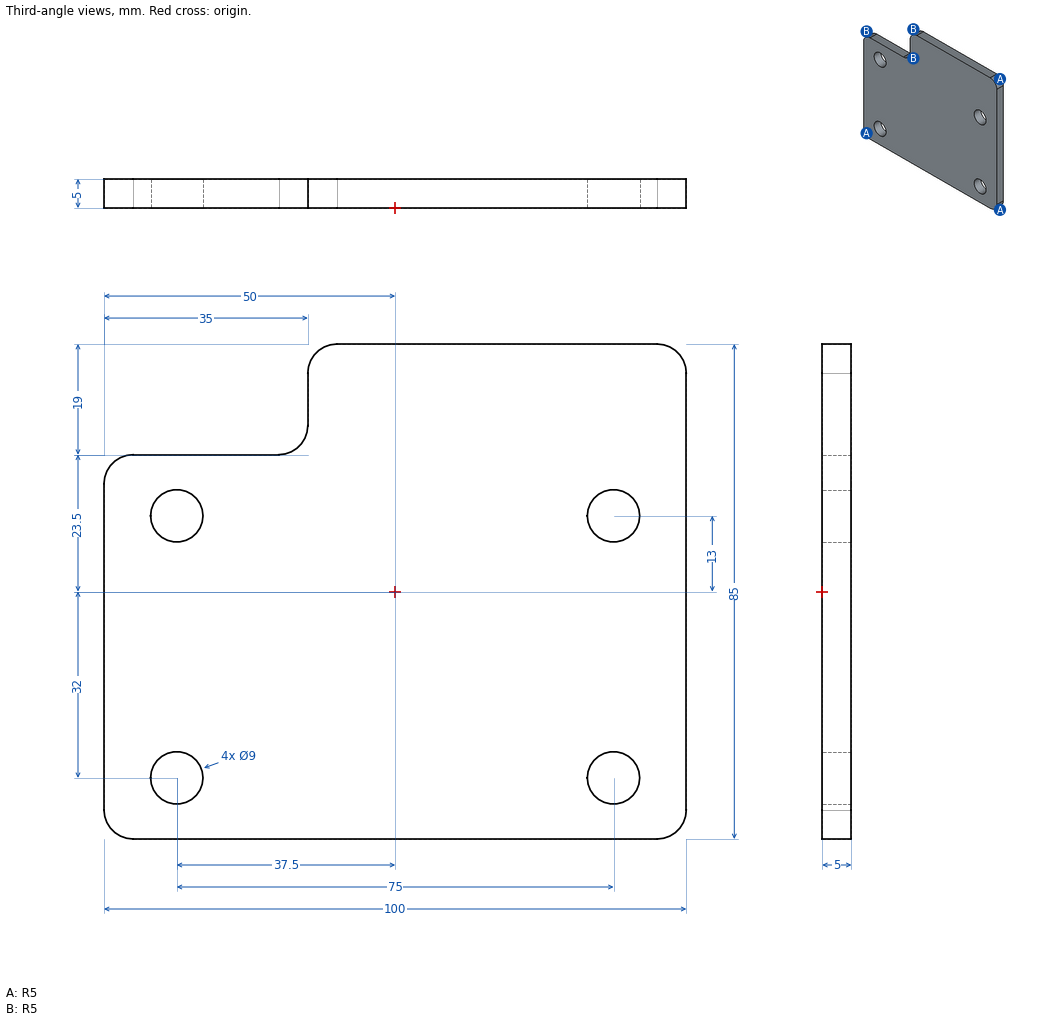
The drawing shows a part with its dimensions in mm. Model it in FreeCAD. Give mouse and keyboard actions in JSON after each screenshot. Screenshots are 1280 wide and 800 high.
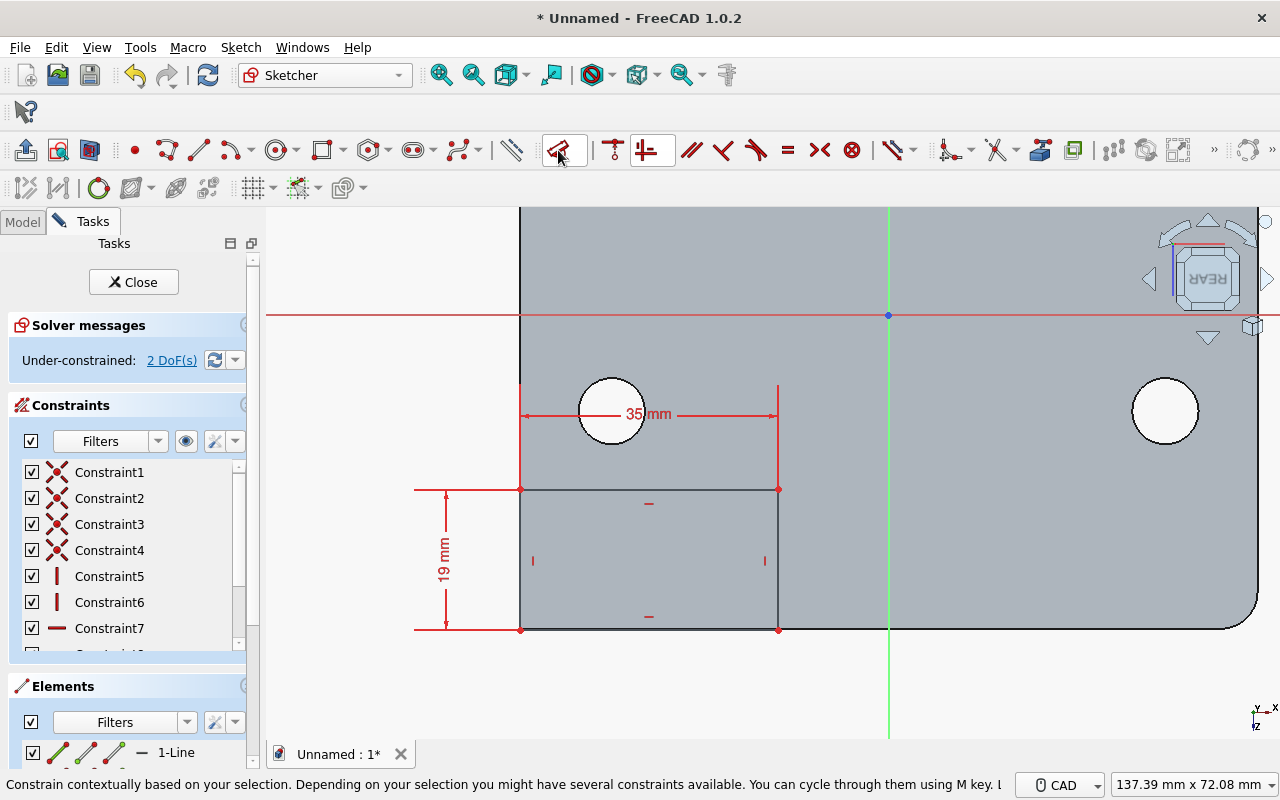
{"action": "left_click", "coordinate": [520, 490]}
{"action": "left_click", "coordinate": [704, 281]}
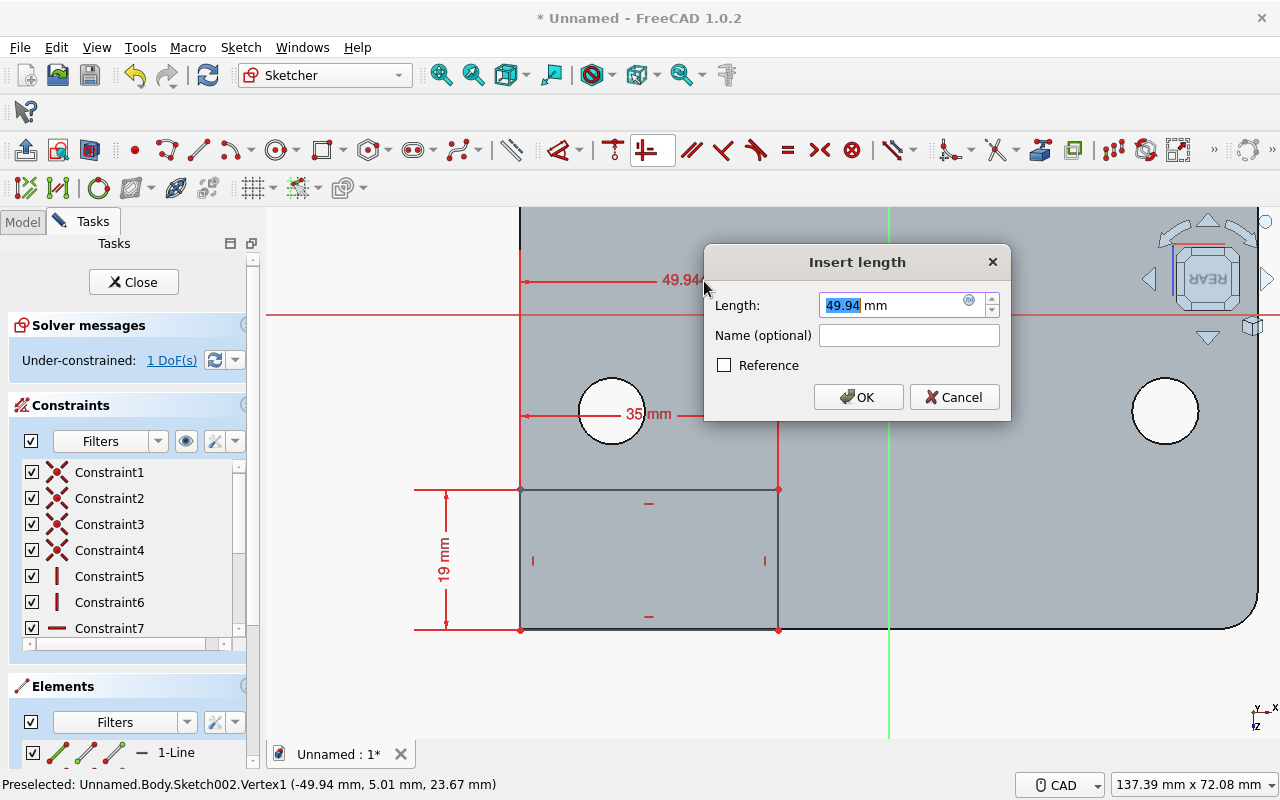
{"action": "type", "text": "50"}
{"action": "key", "text": "Return"}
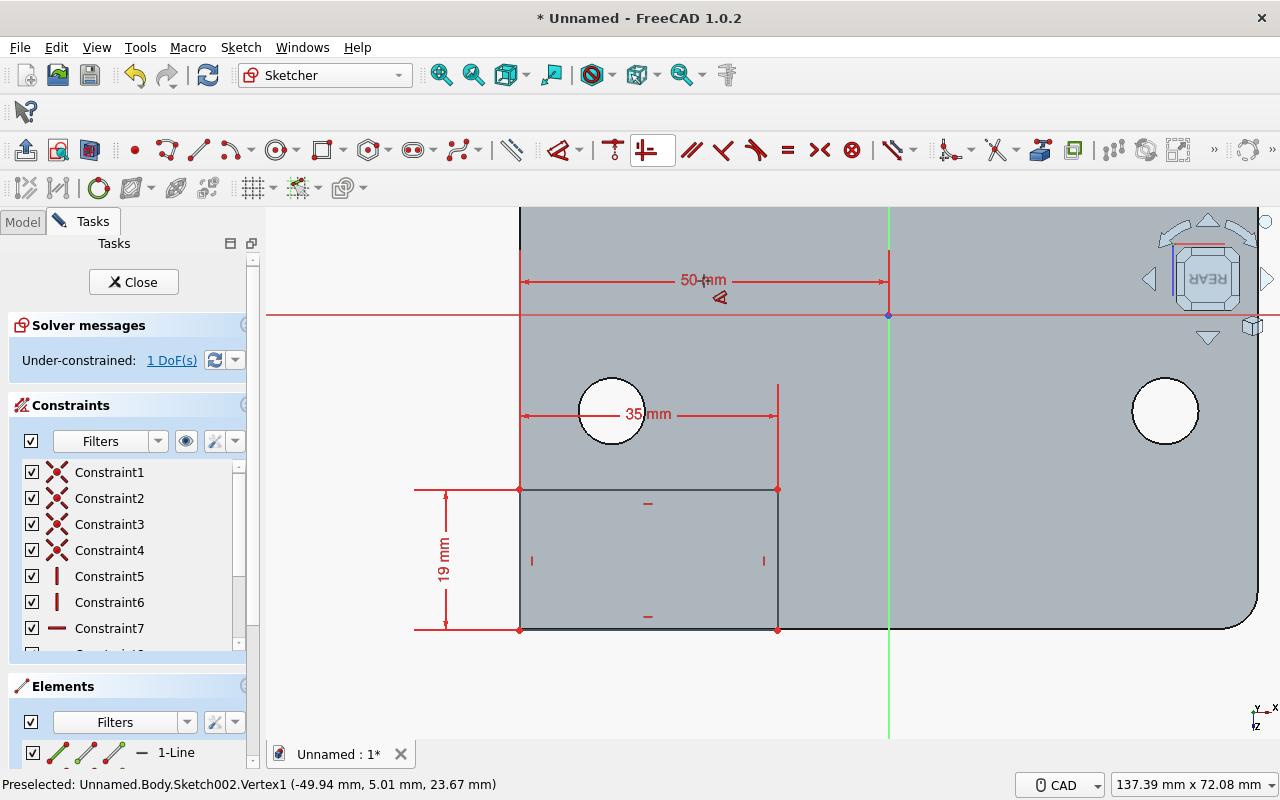
{"action": "left_click", "coordinate": [520, 490]}
{"action": "left_click", "coordinate": [923, 403]}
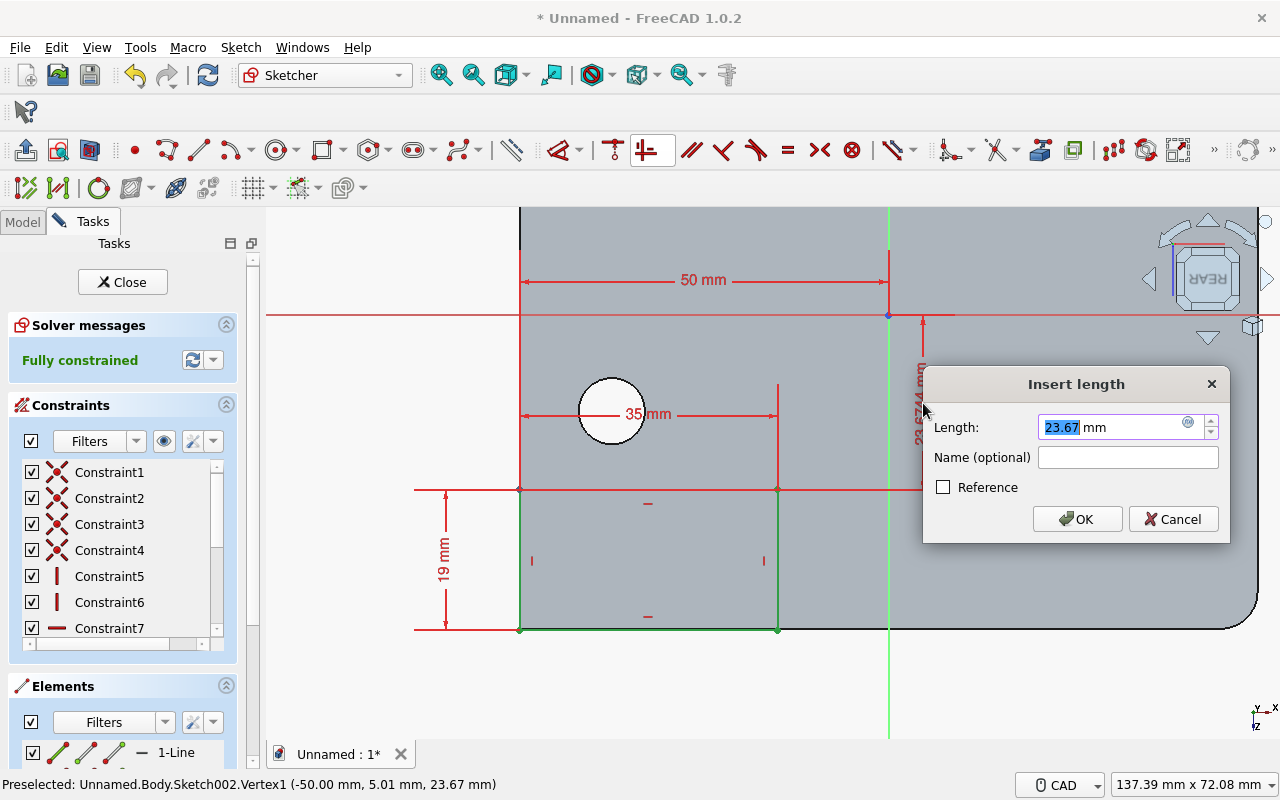
{"action": "type", "text": "23.5"}
{"action": "key", "text": "Return"}
{"action": "key", "text": "Escape"}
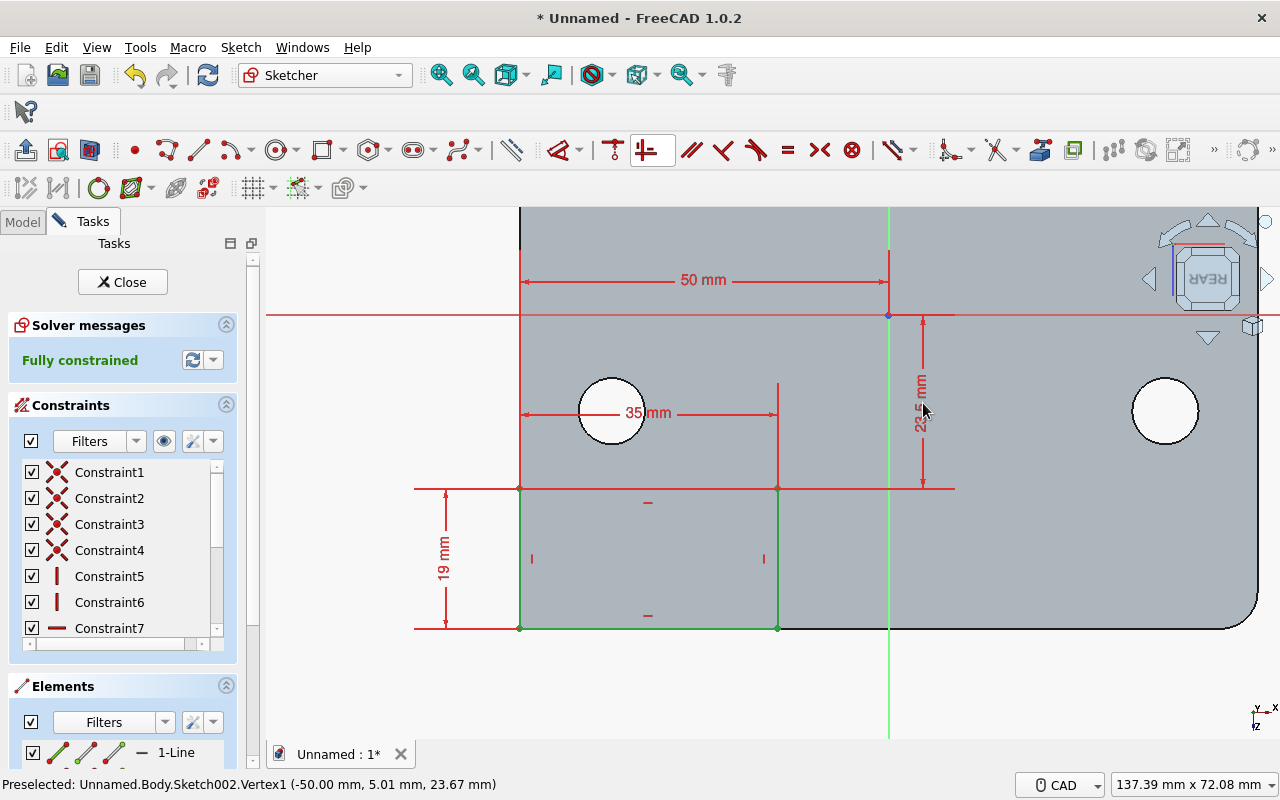
{"action": "left_click", "coordinate": [123, 282]}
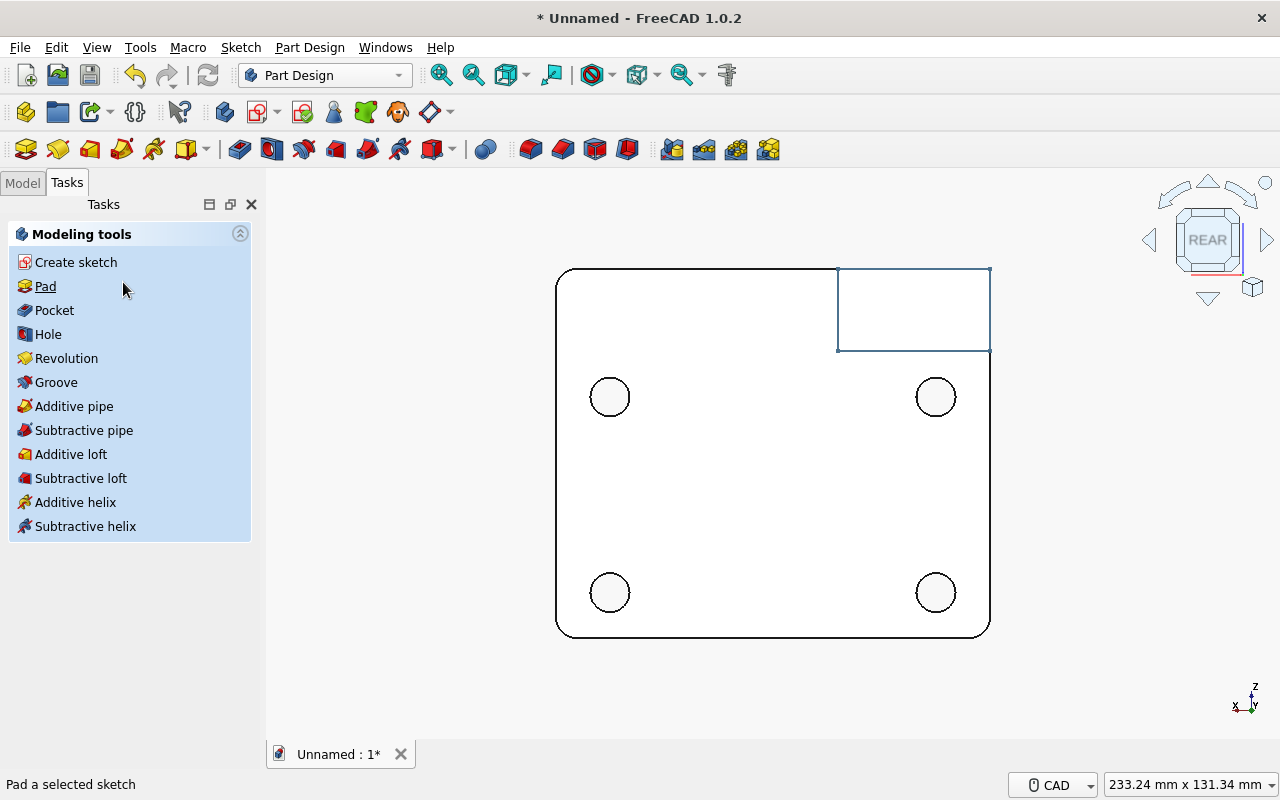
{"action": "left_click", "coordinate": [240, 150]}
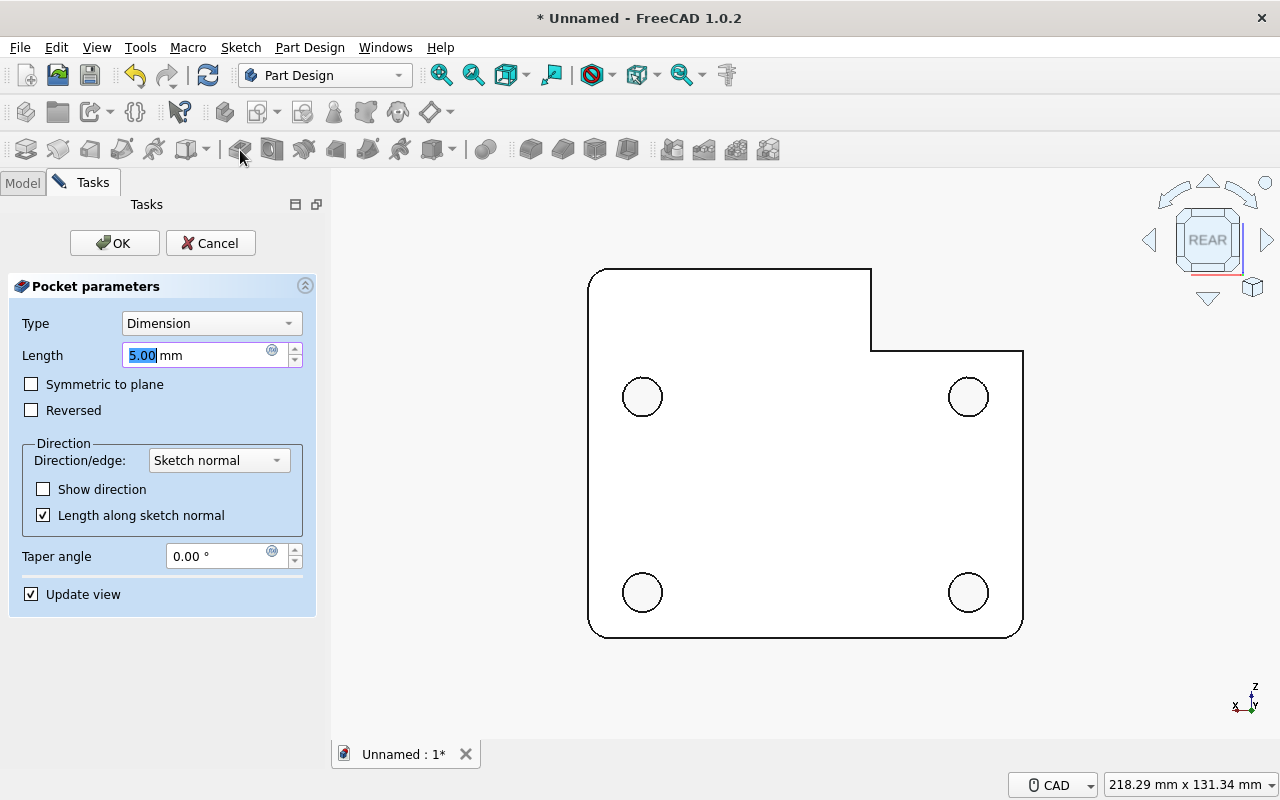
{"action": "type", "text": "5"}
{"action": "key", "text": "Tab"}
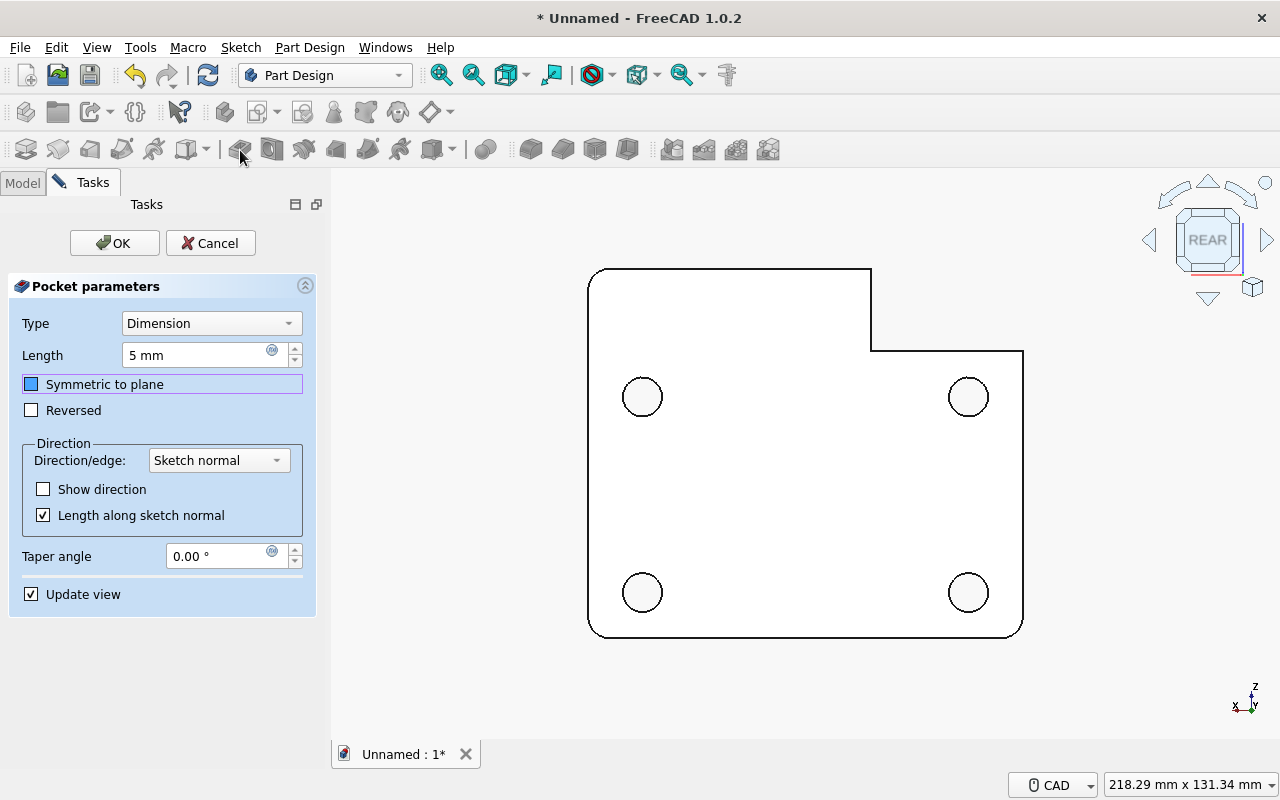
{"action": "left_click", "coordinate": [115, 243]}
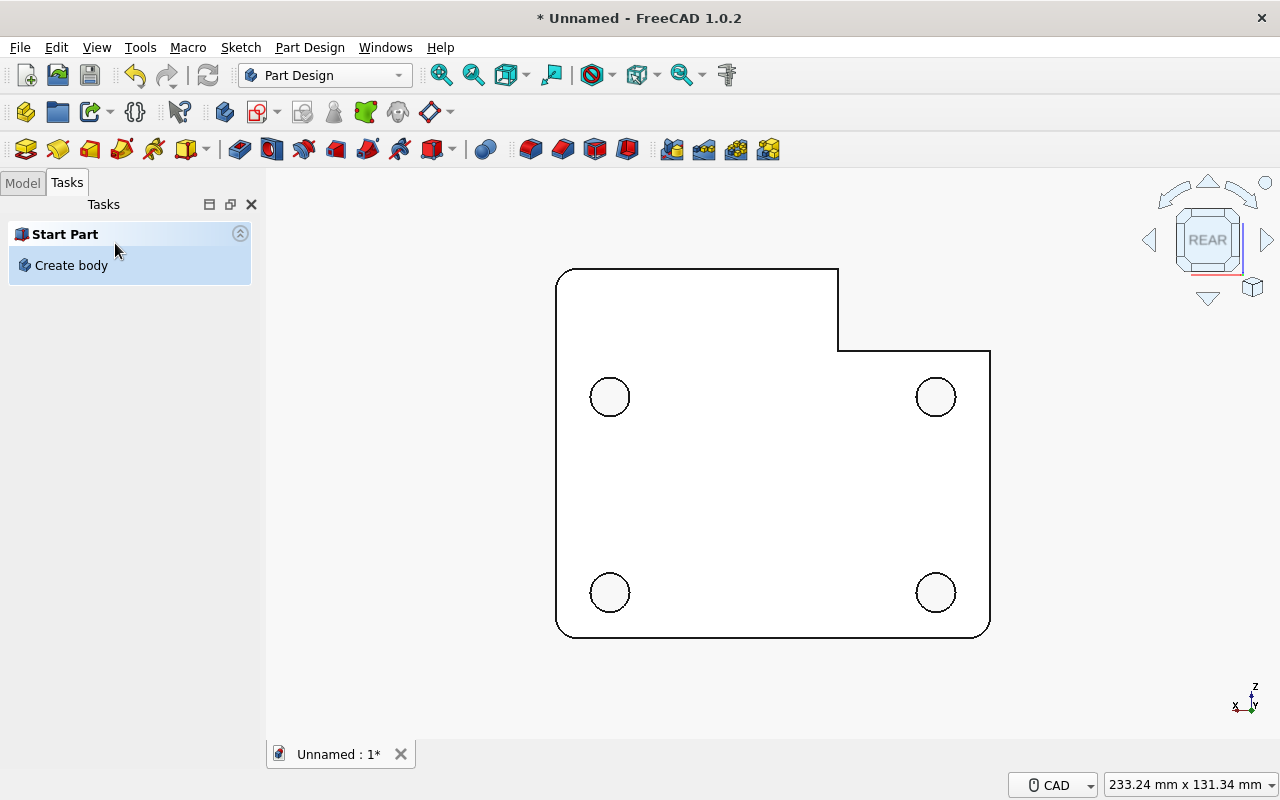
{"action": "scroll", "coordinate": [990, 350], "scroll_direction": "up", "scroll_amount": 4}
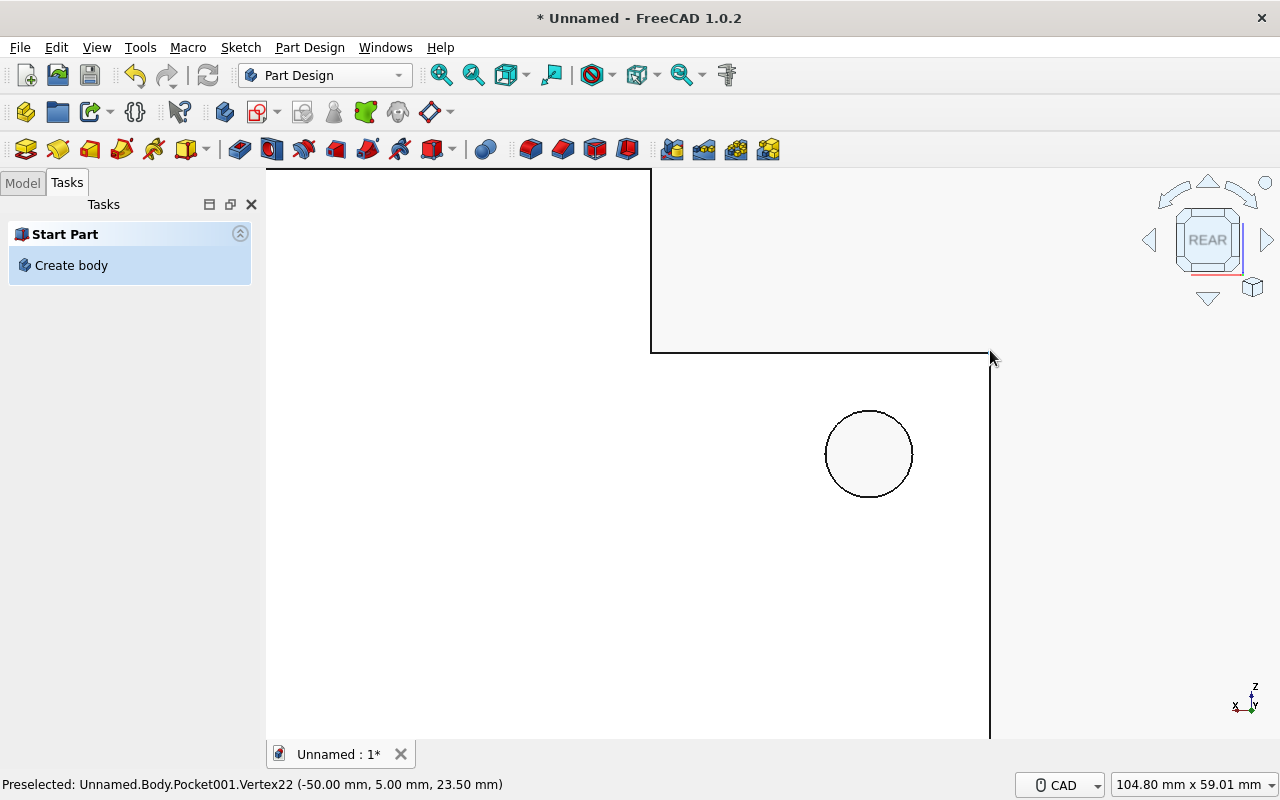
{"action": "left_click", "coordinate": [442, 76]}